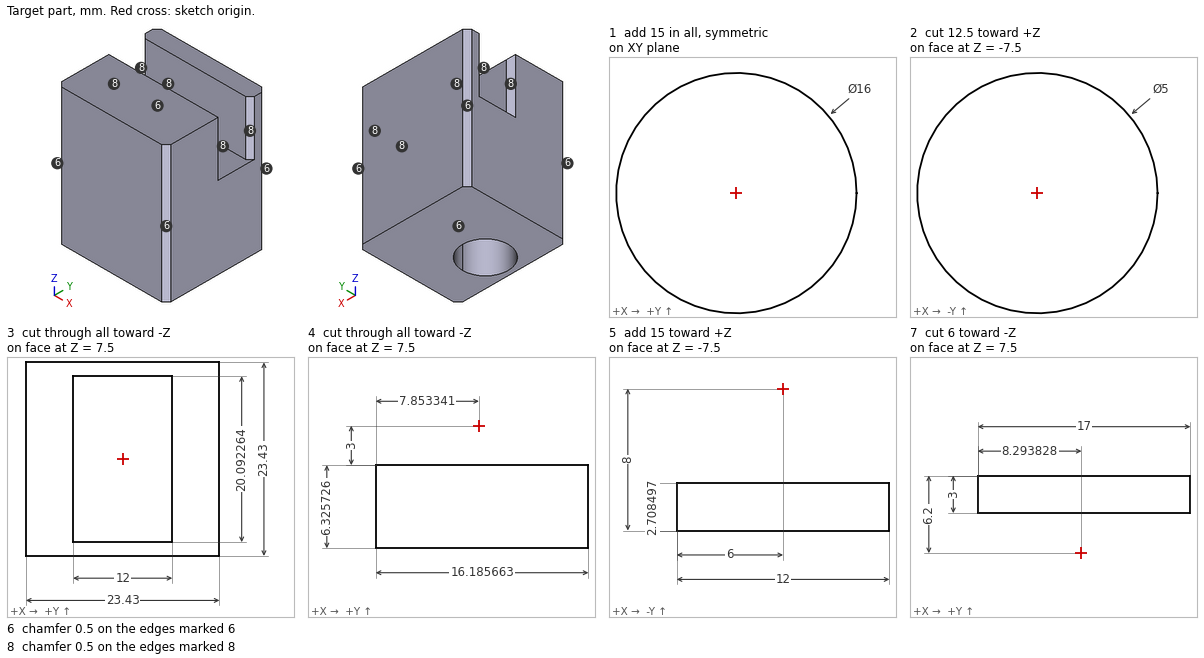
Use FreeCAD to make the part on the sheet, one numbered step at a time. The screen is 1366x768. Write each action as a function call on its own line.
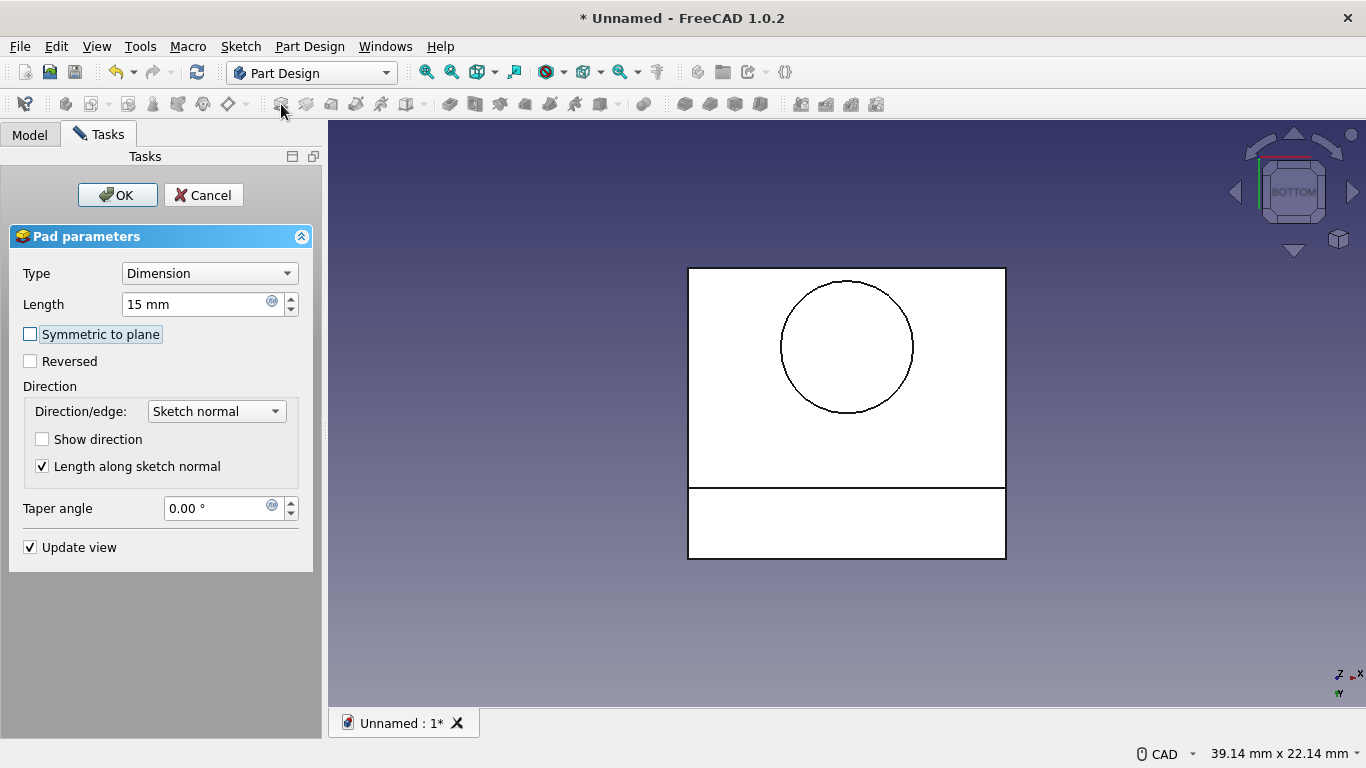
click(31, 361)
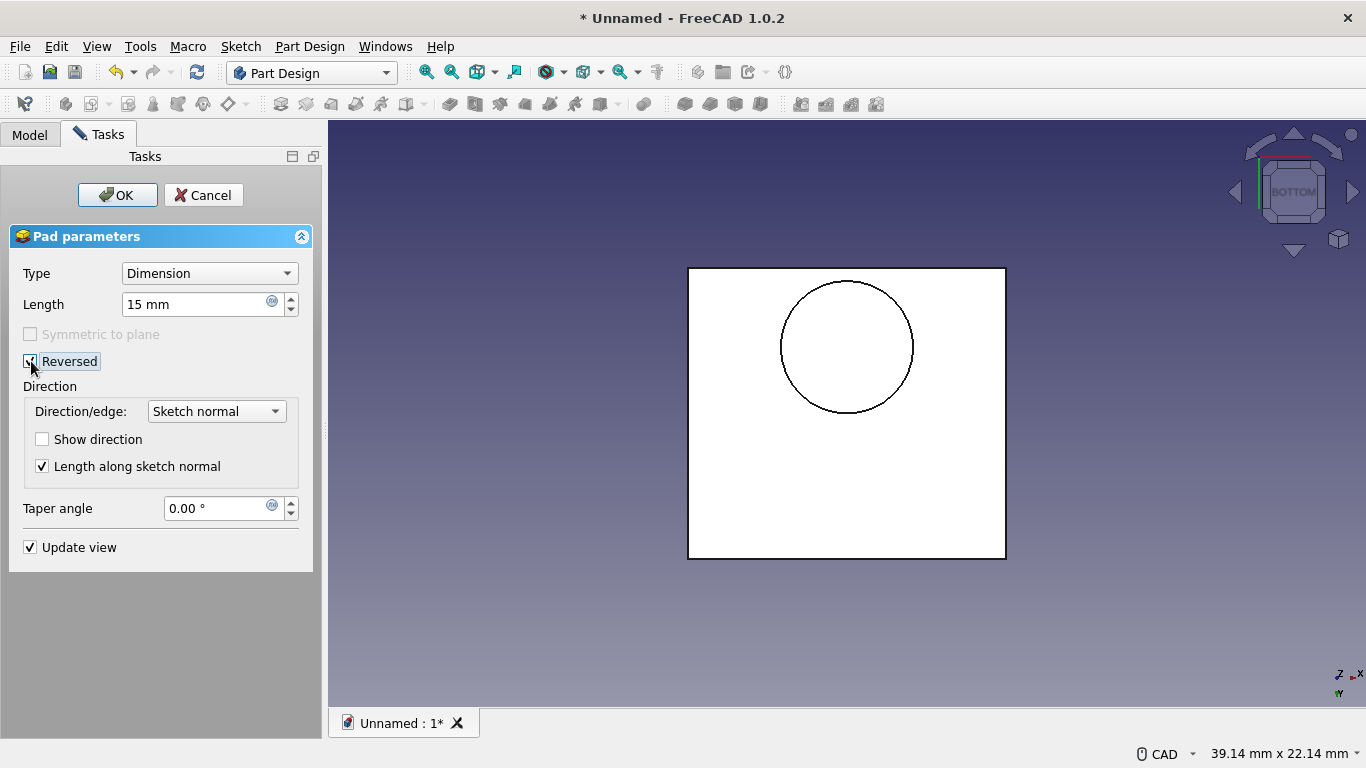
click(118, 195)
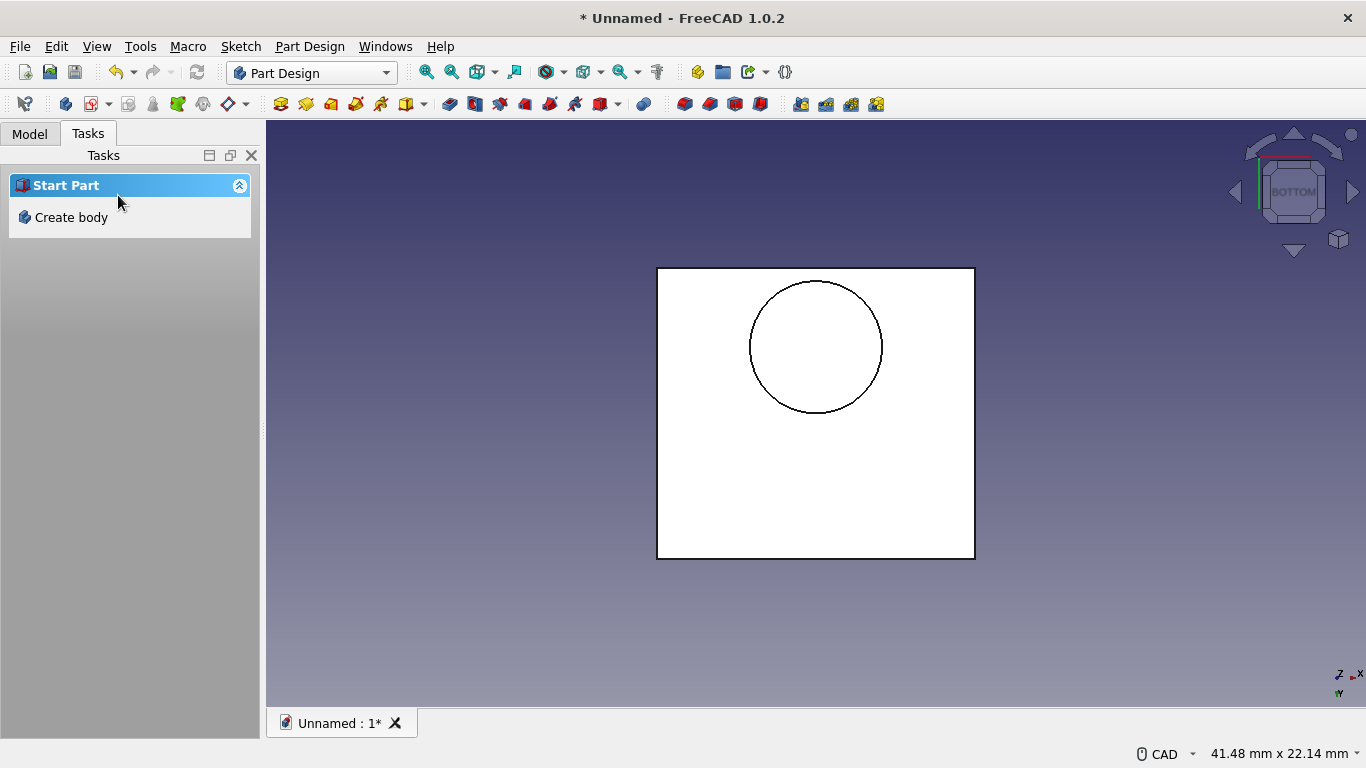
key(0)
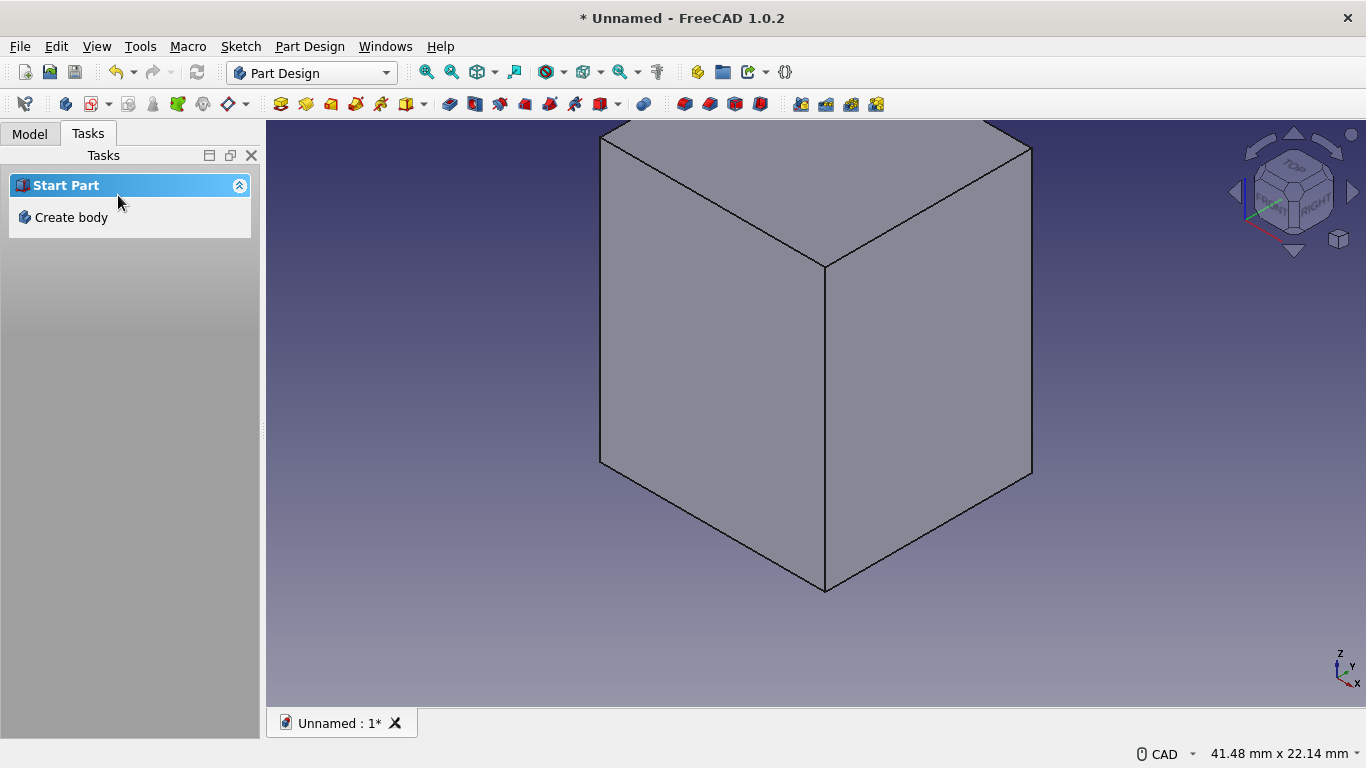
click(427, 72)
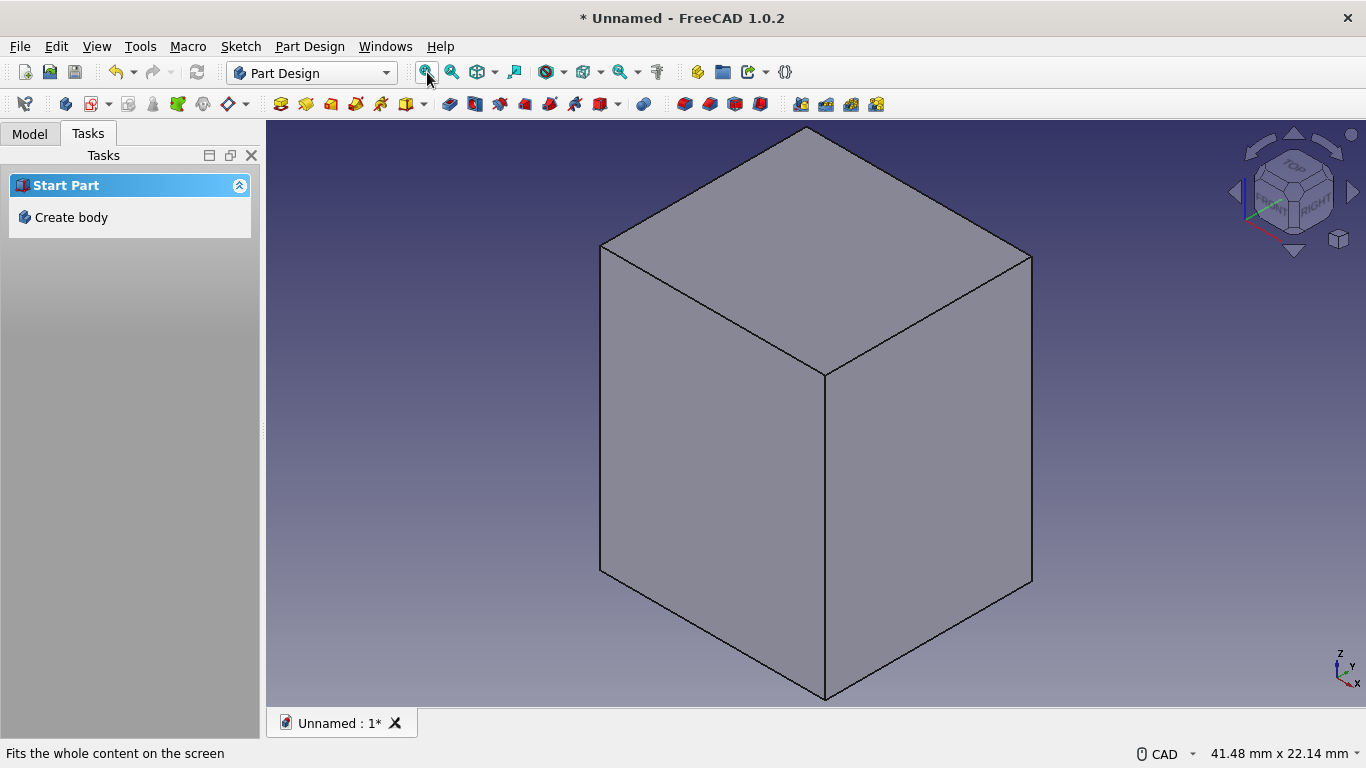
click(825, 537)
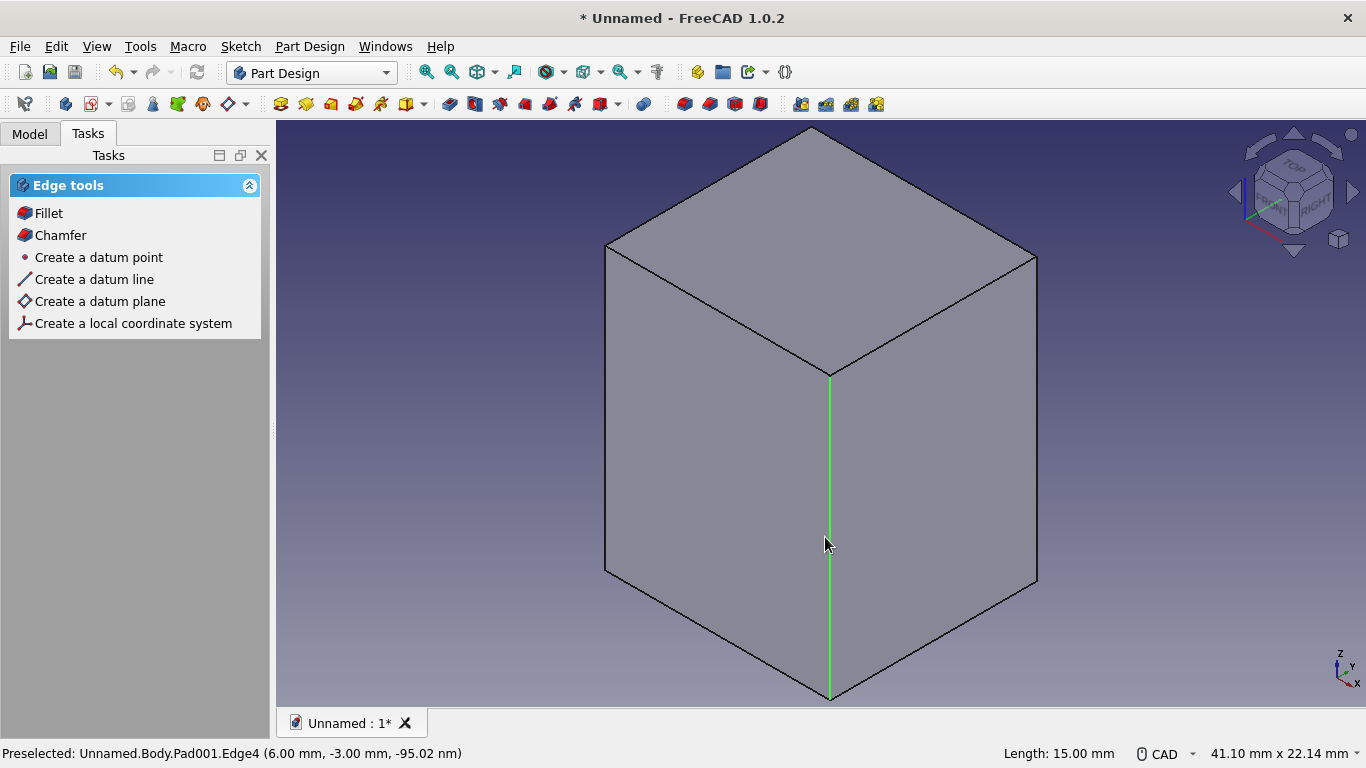
key(2)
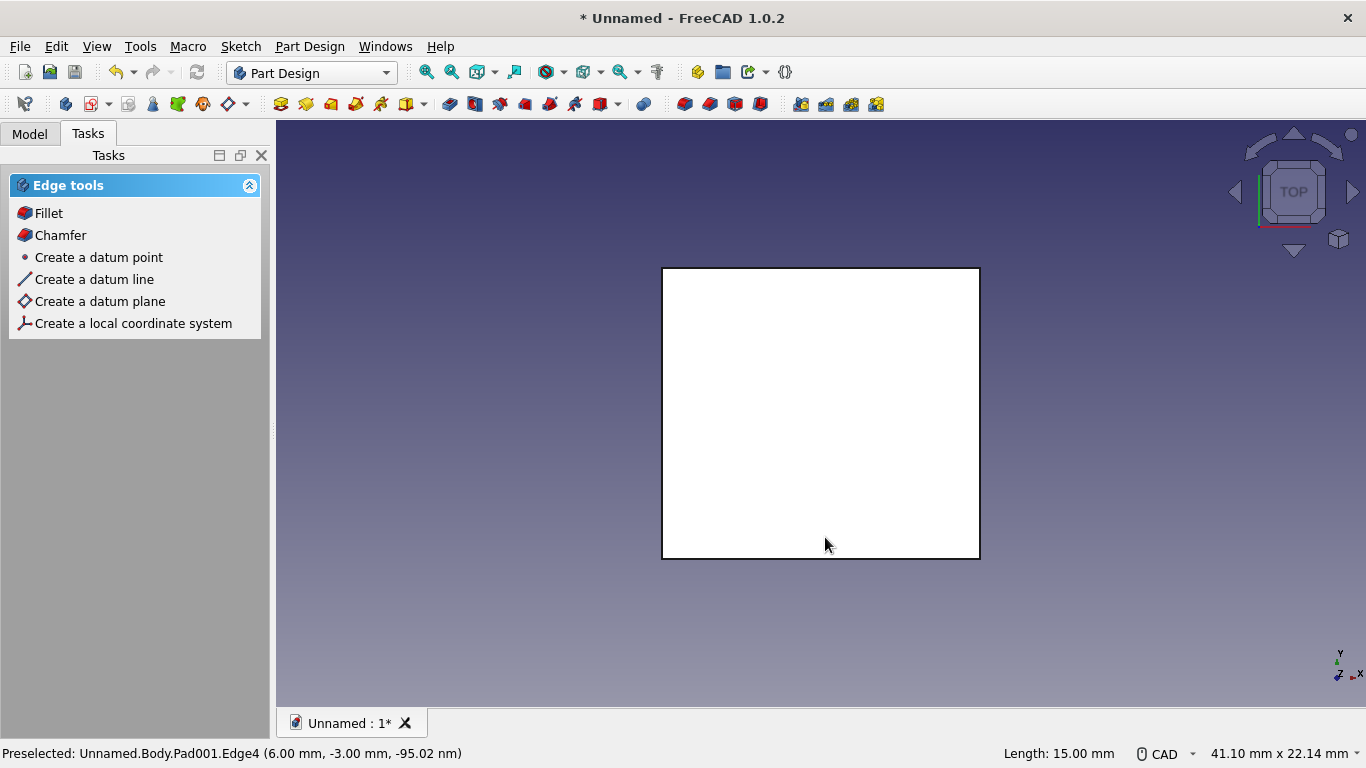
key(1)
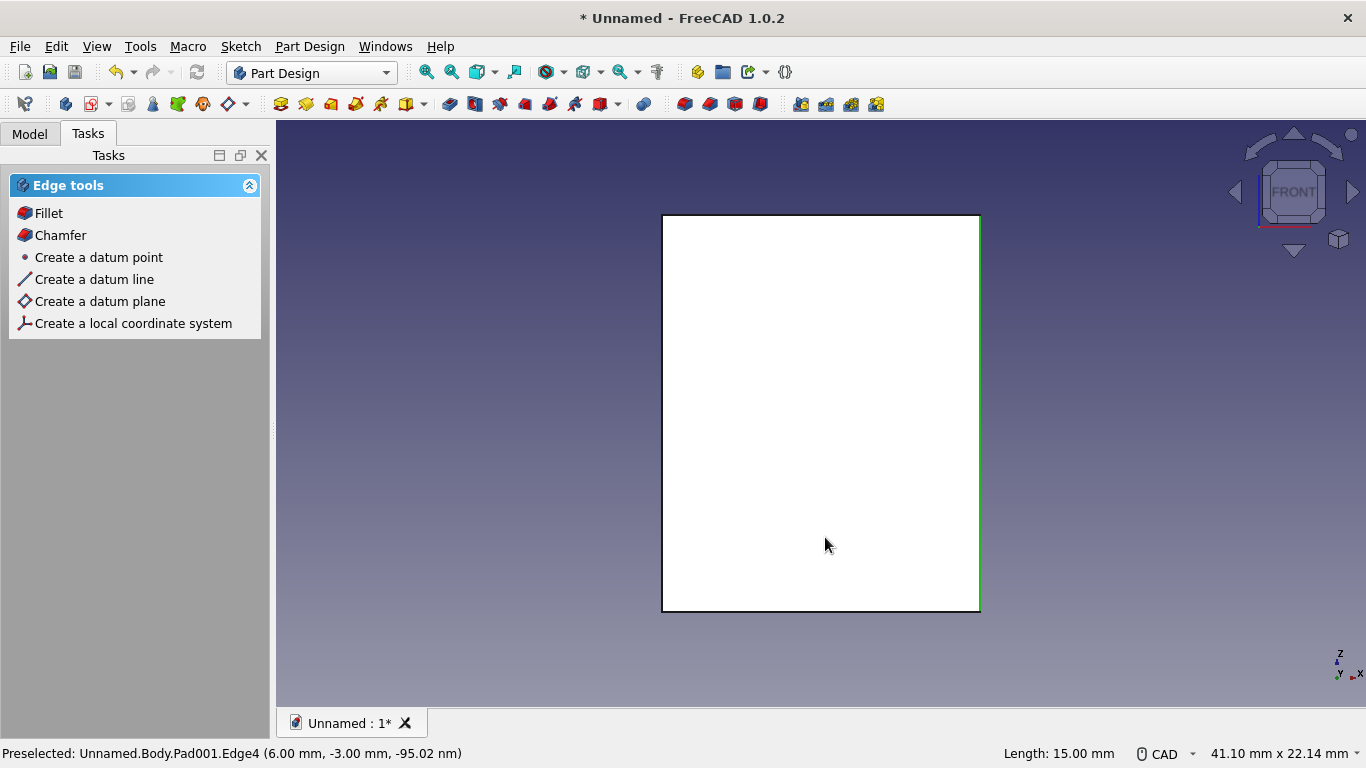
click(662, 412, ctrl)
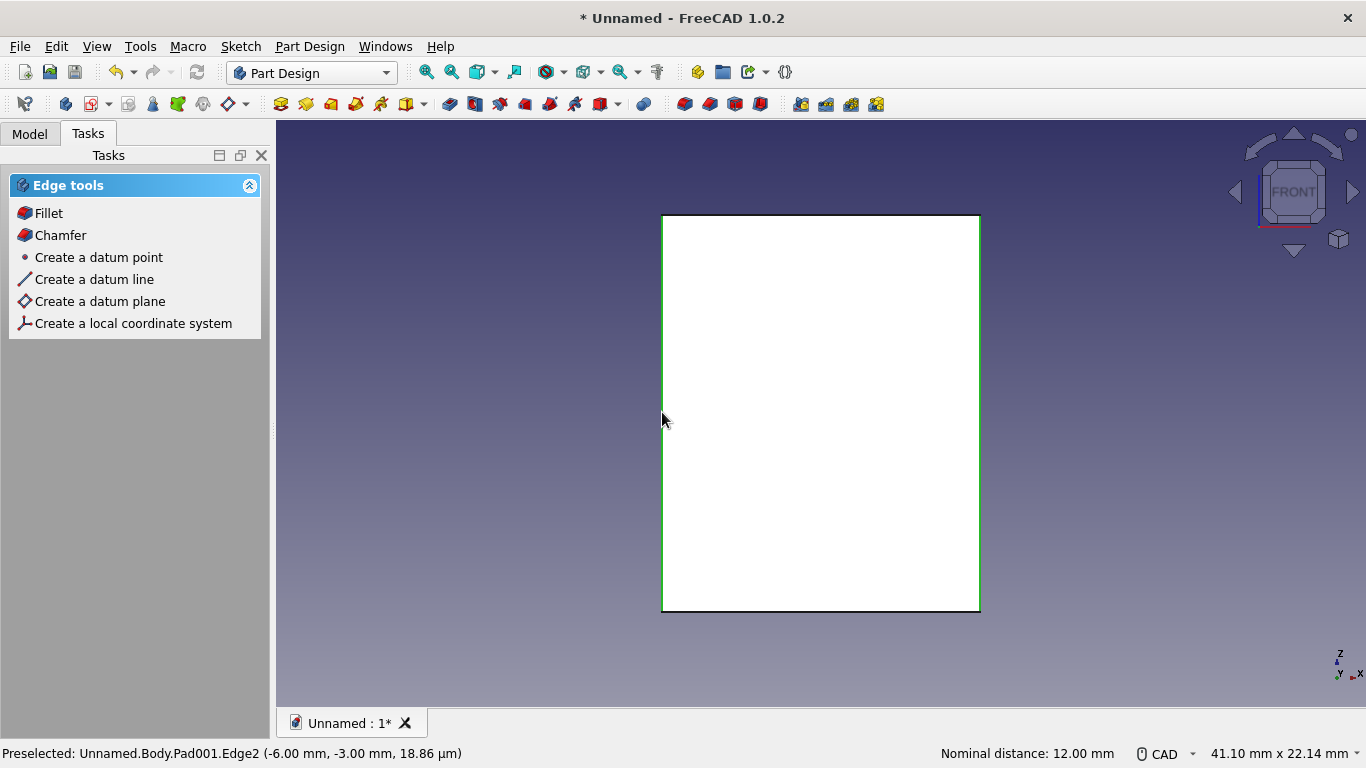
key(3)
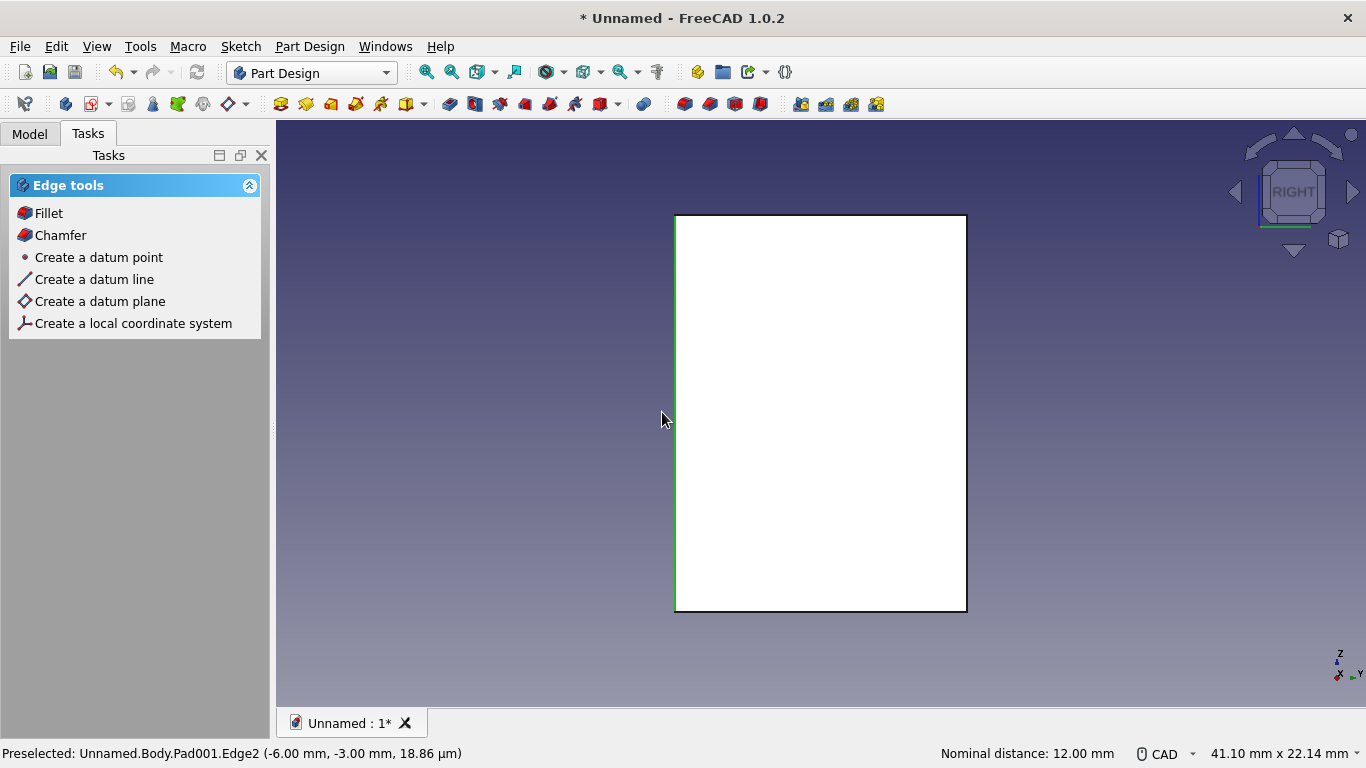
click(967, 412, ctrl)